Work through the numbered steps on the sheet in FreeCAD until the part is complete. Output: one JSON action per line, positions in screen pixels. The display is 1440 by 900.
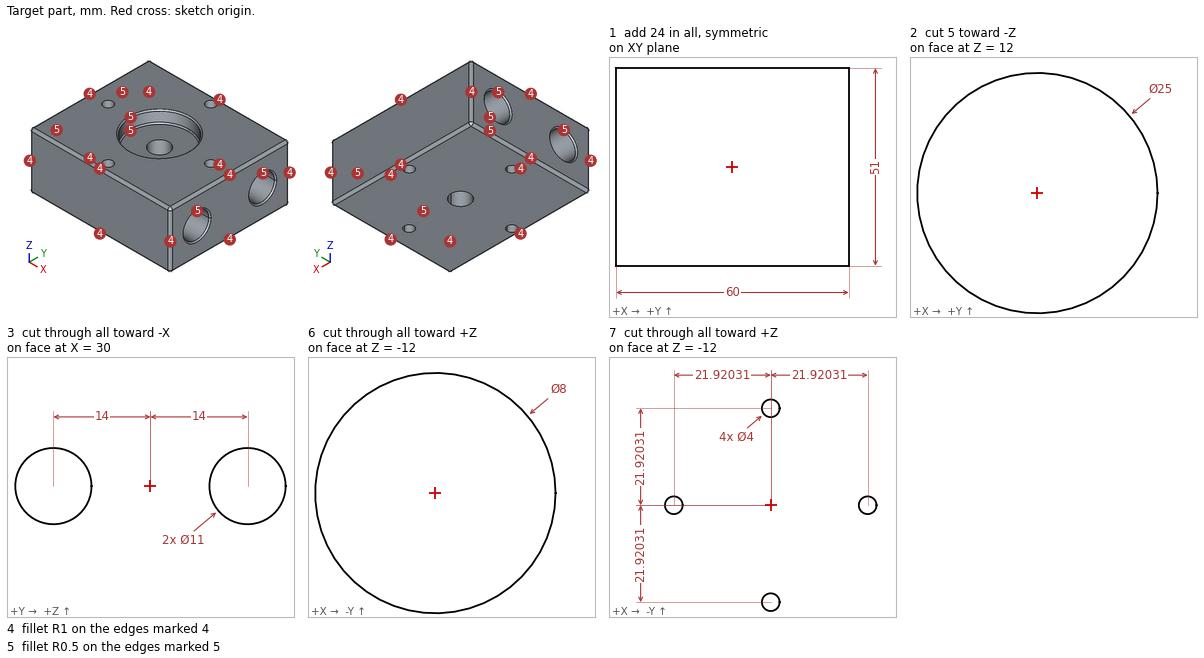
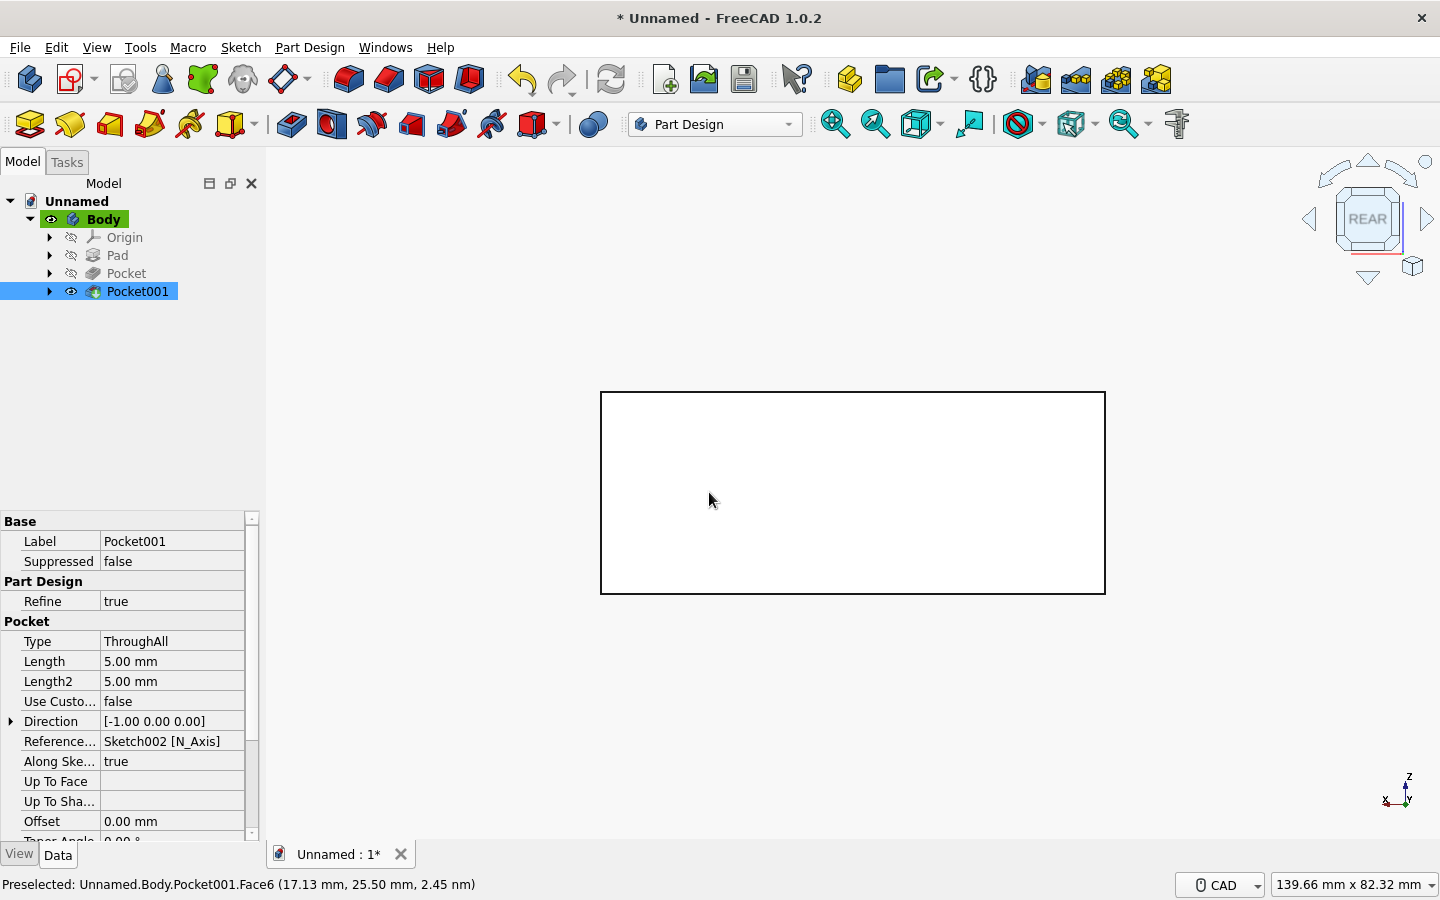
{"action": "left_click", "coordinate": [350, 80]}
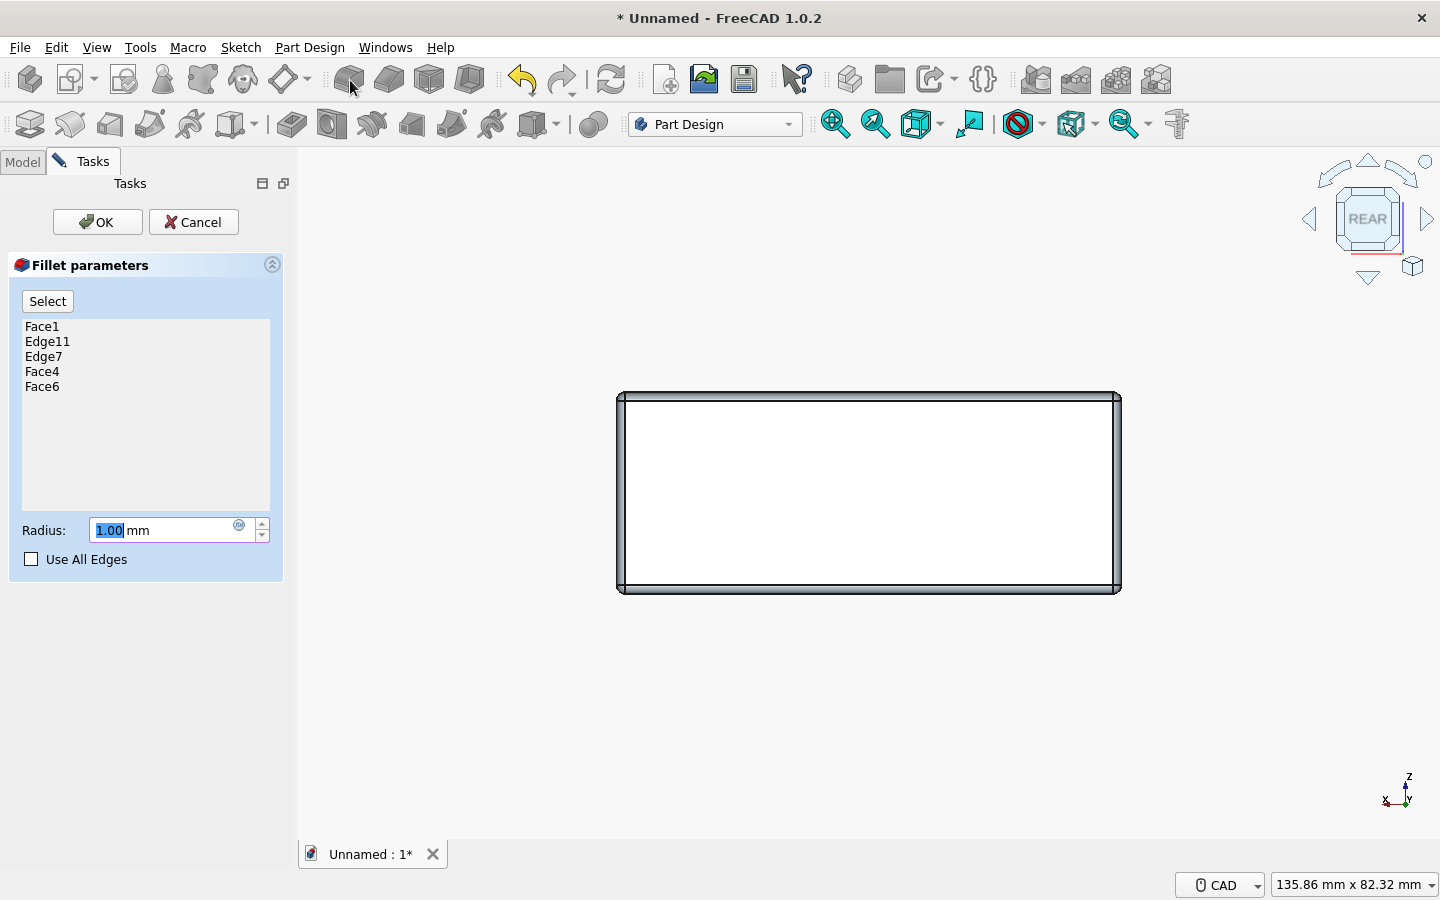
{"action": "type", "text": "1"}
{"action": "key", "text": "Tab"}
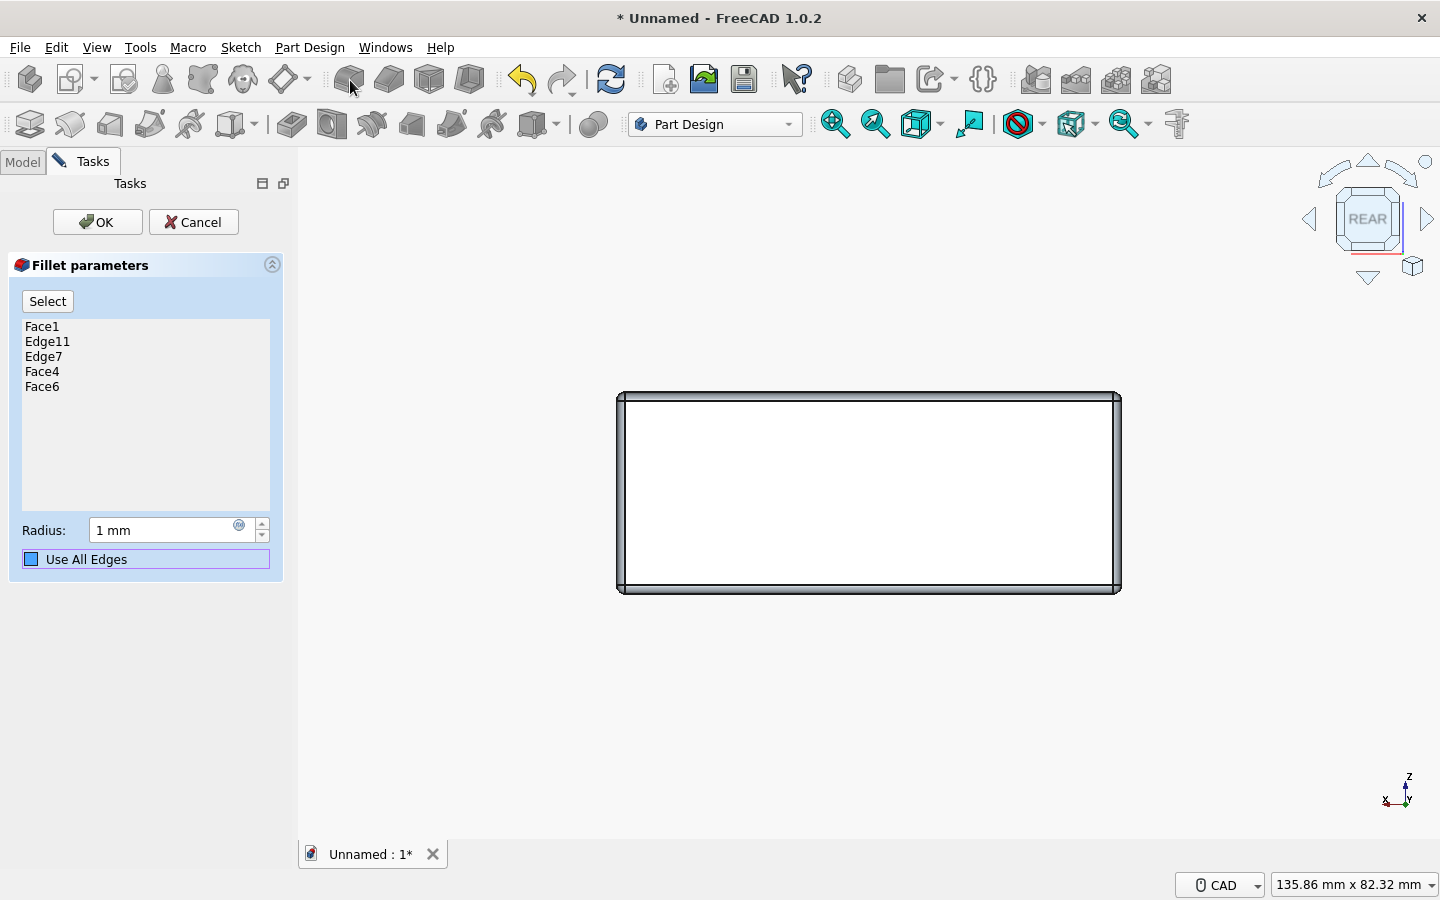
{"action": "left_click", "coordinate": [98, 222]}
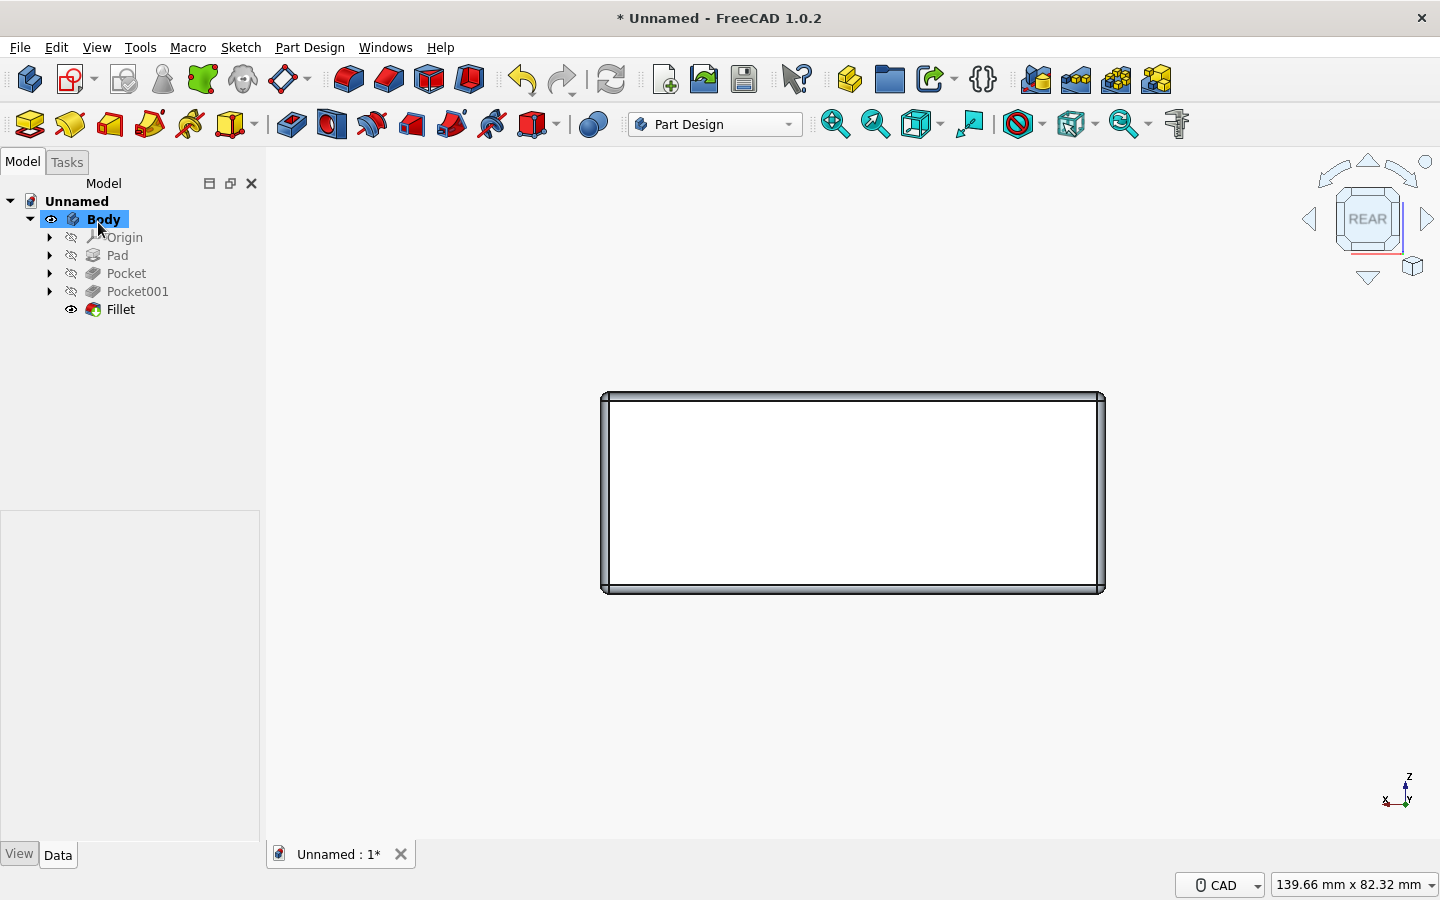
{"action": "left_click", "coordinate": [836, 124]}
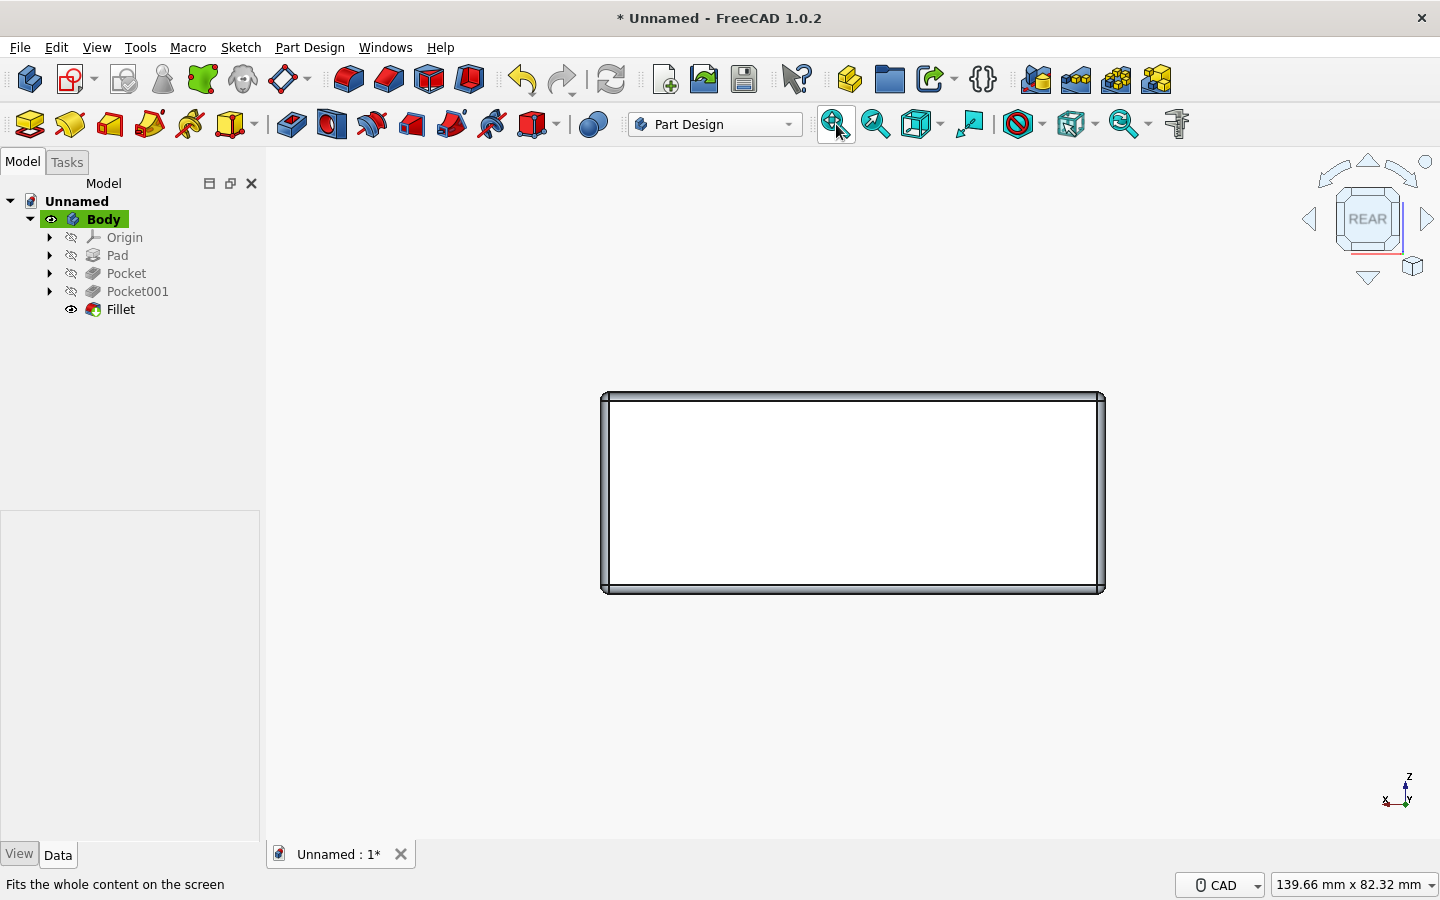
{"action": "key", "text": "0"}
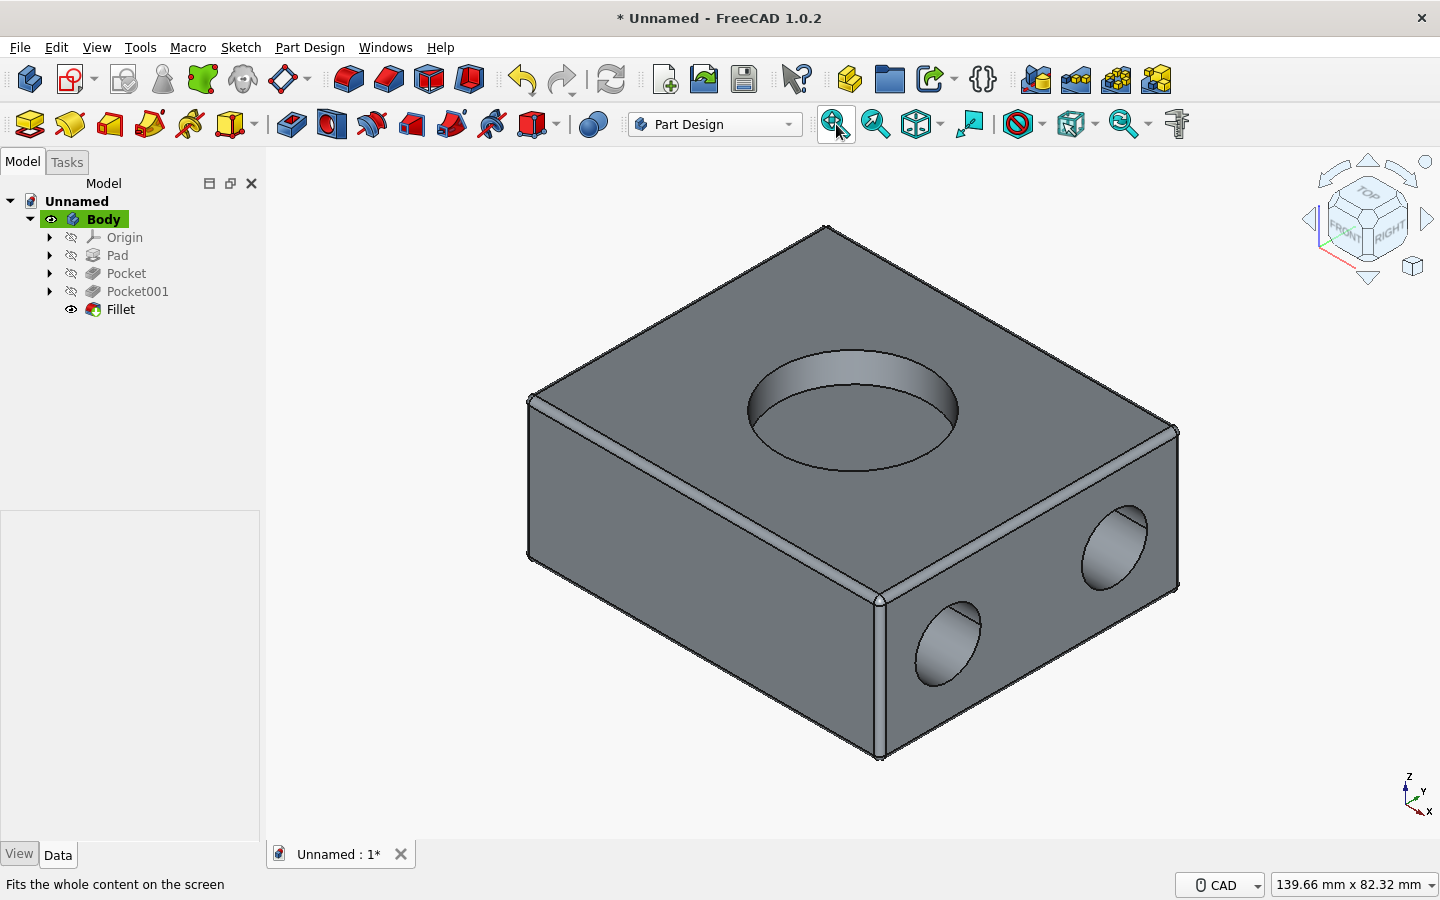
{"action": "left_click", "coordinate": [779, 367]}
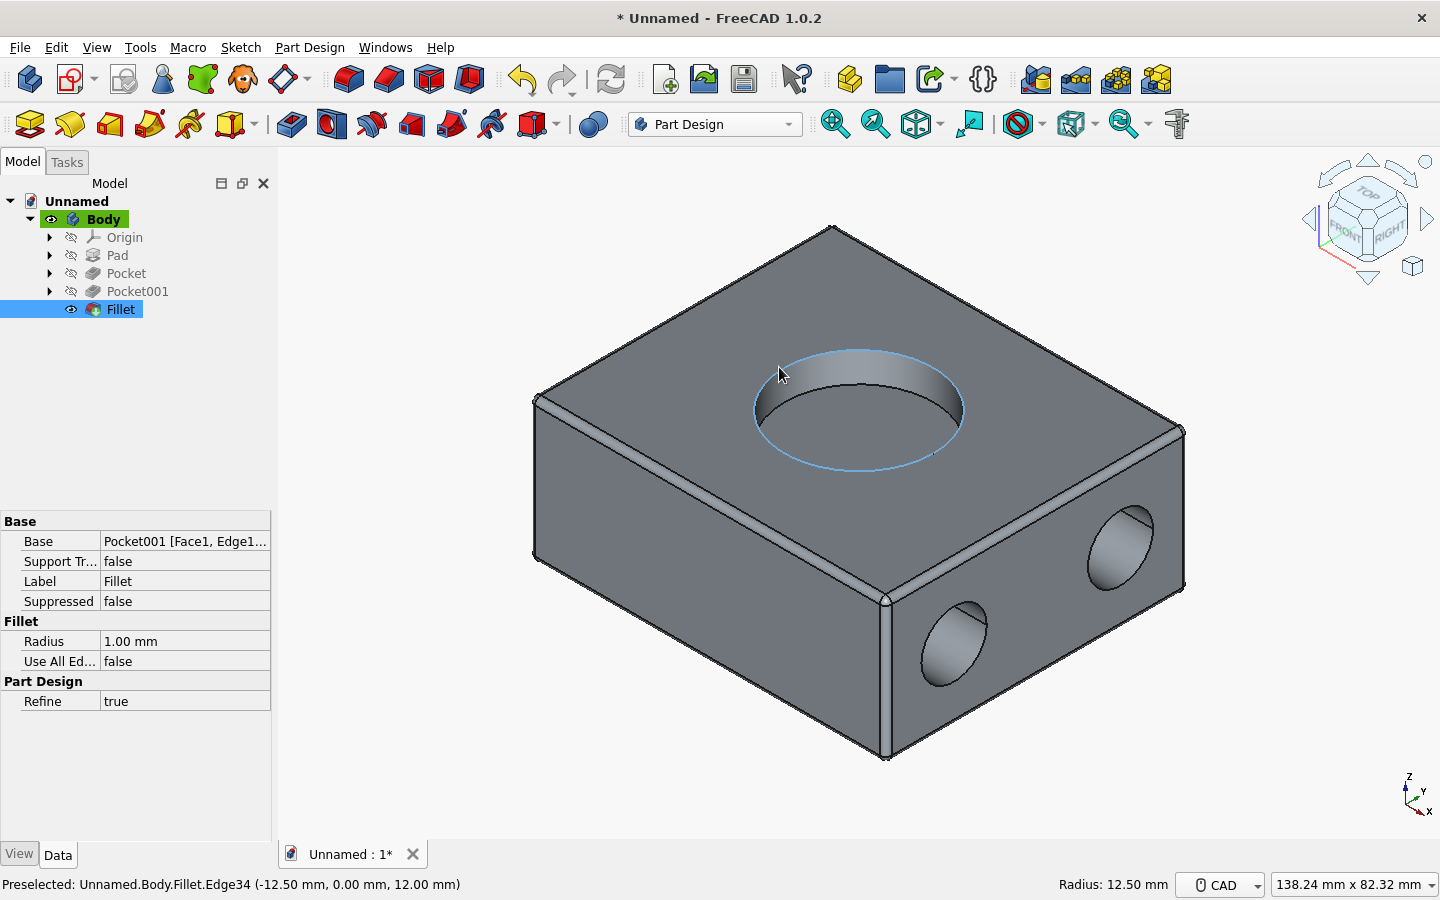
{"action": "left_click", "coordinate": [1110, 589], "text": "ctrl"}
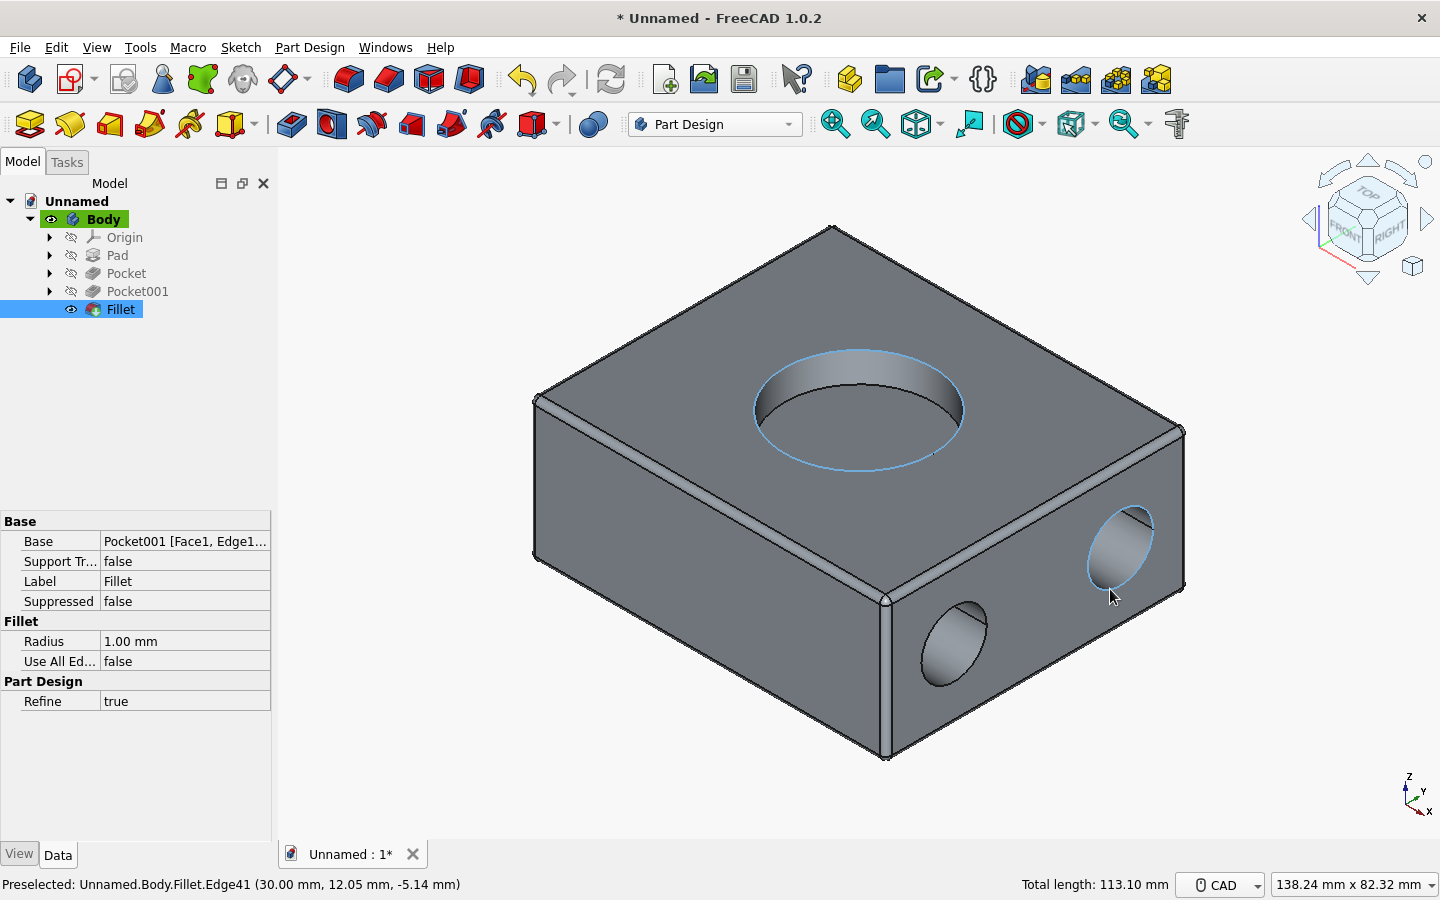
{"action": "left_click", "coordinate": [944, 685], "text": "ctrl"}